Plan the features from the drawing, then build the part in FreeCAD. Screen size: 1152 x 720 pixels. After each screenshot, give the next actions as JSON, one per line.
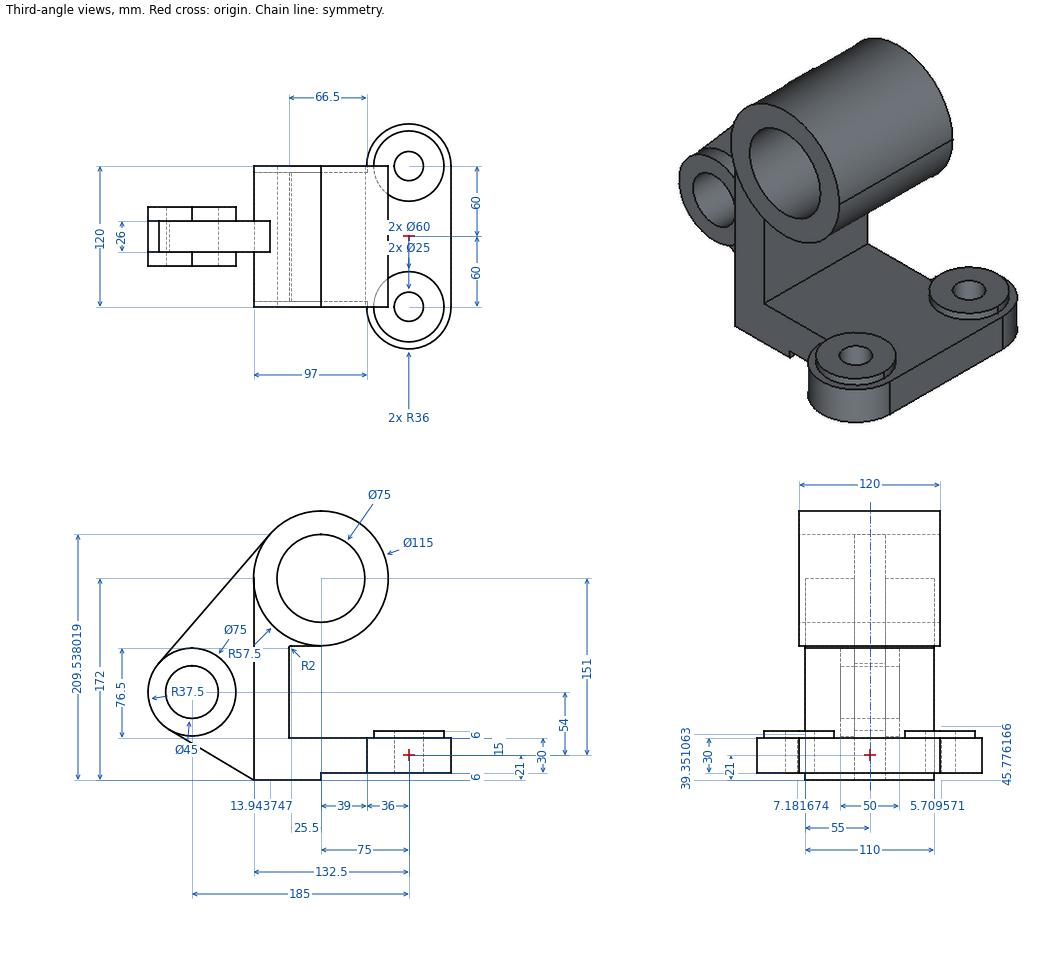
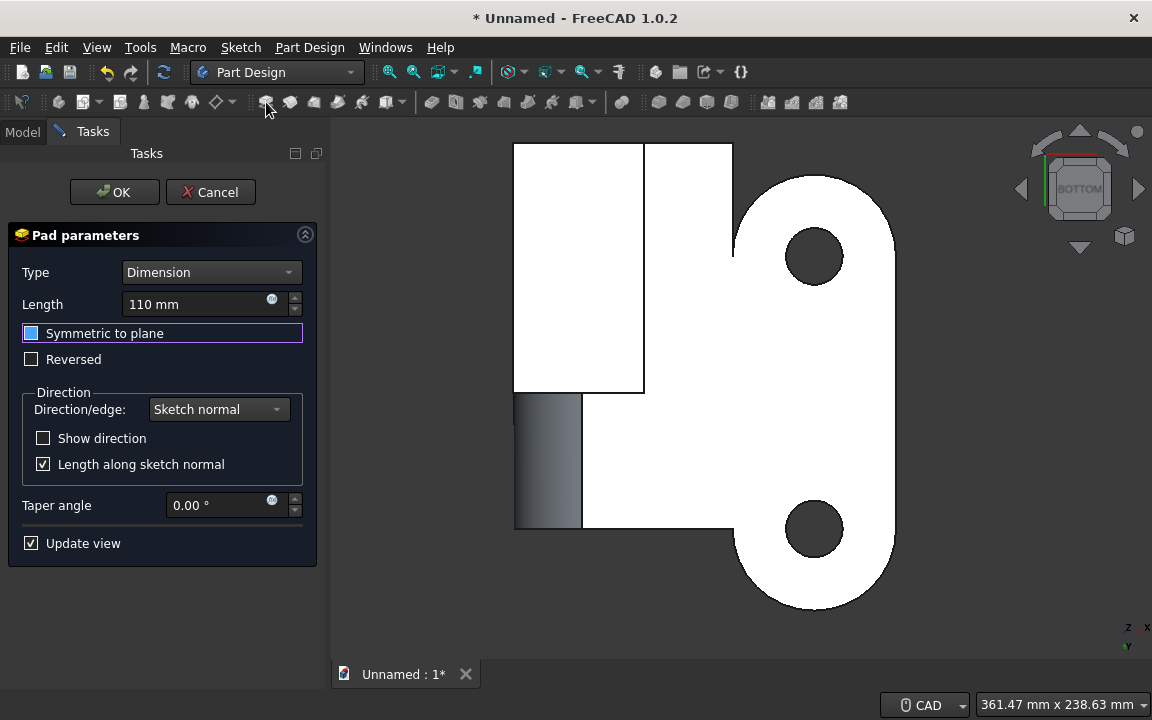
{"action": "left_click", "coordinate": [30, 333]}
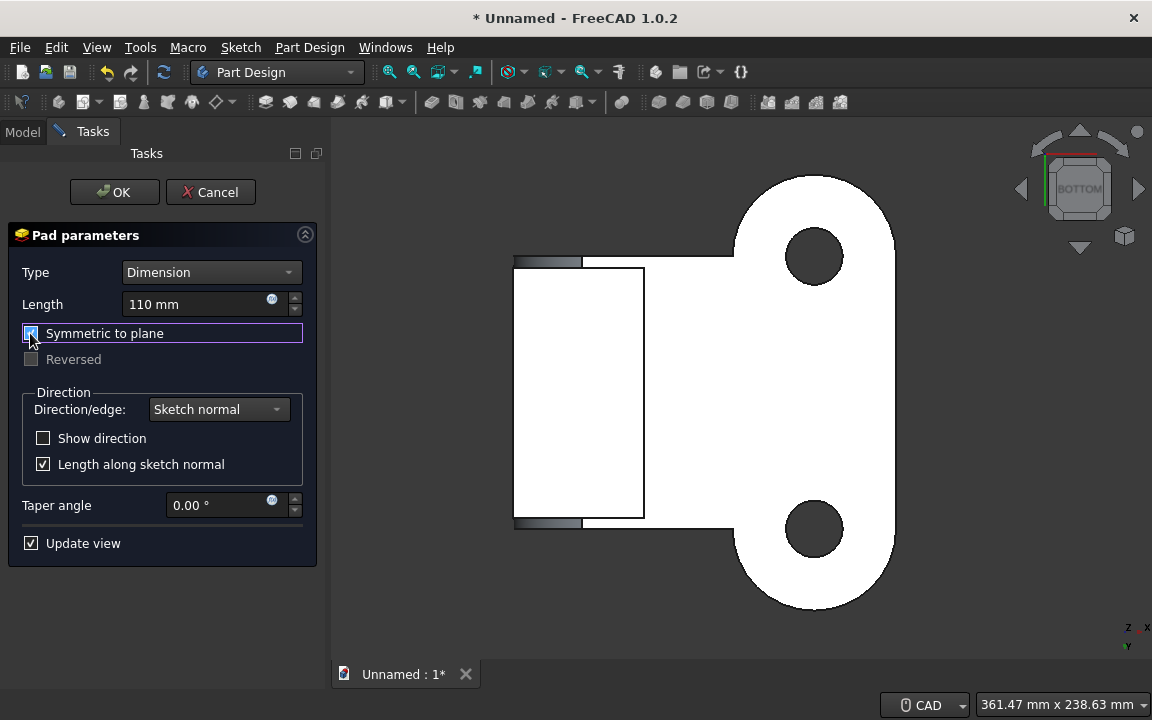
{"action": "left_click", "coordinate": [115, 192]}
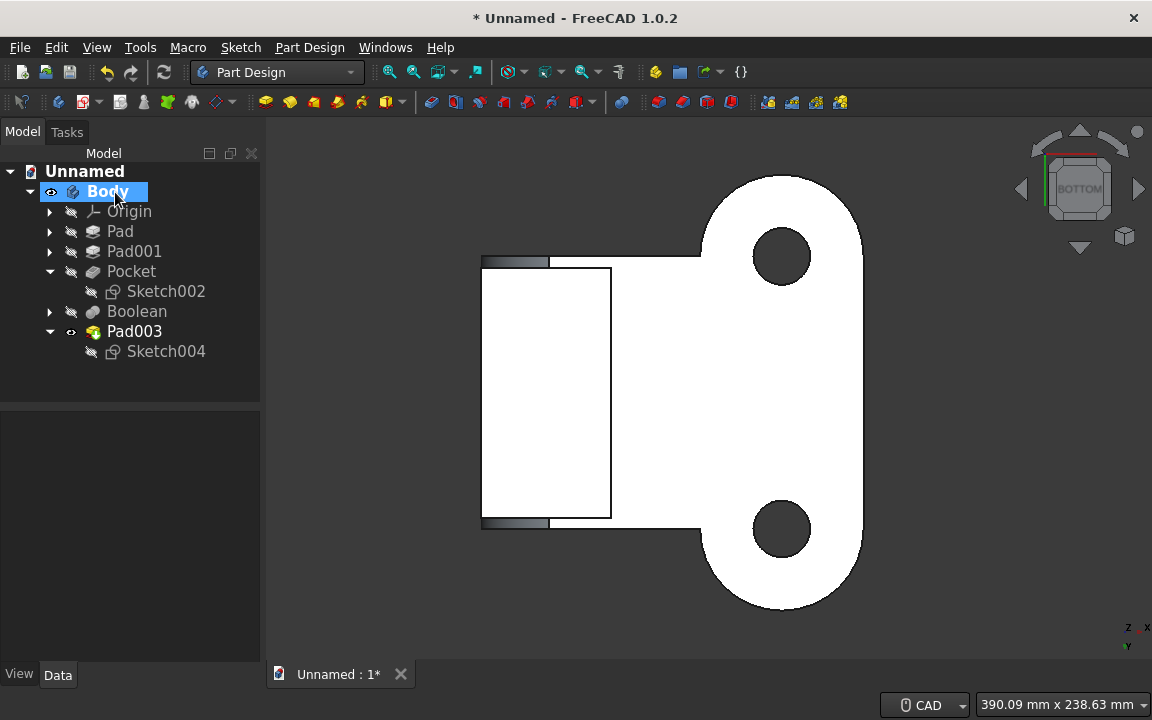
{"action": "key", "text": "6"}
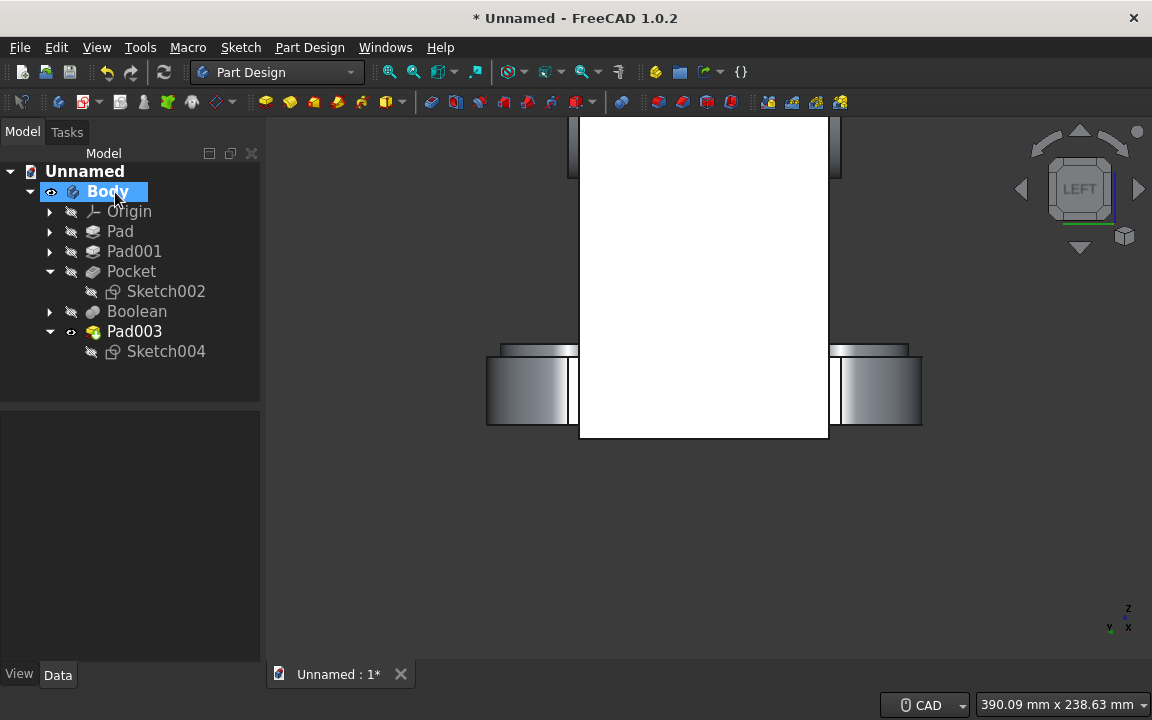
{"action": "key", "text": "v f"}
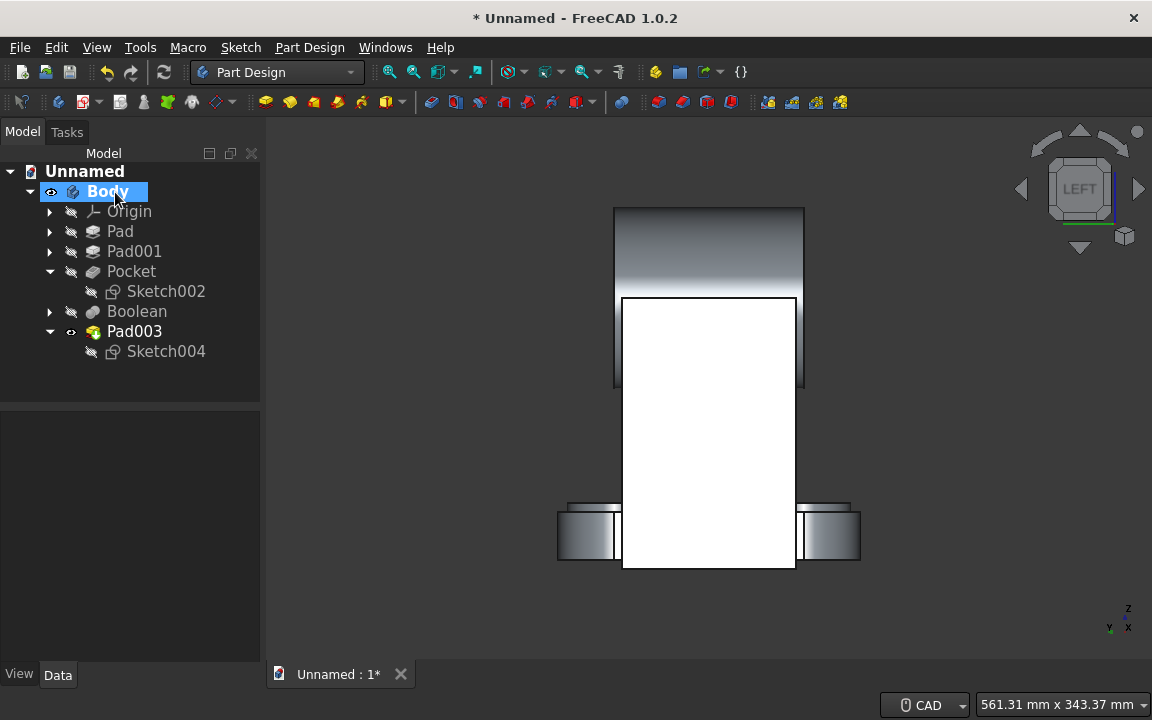
{"action": "left_click", "coordinate": [709, 394]}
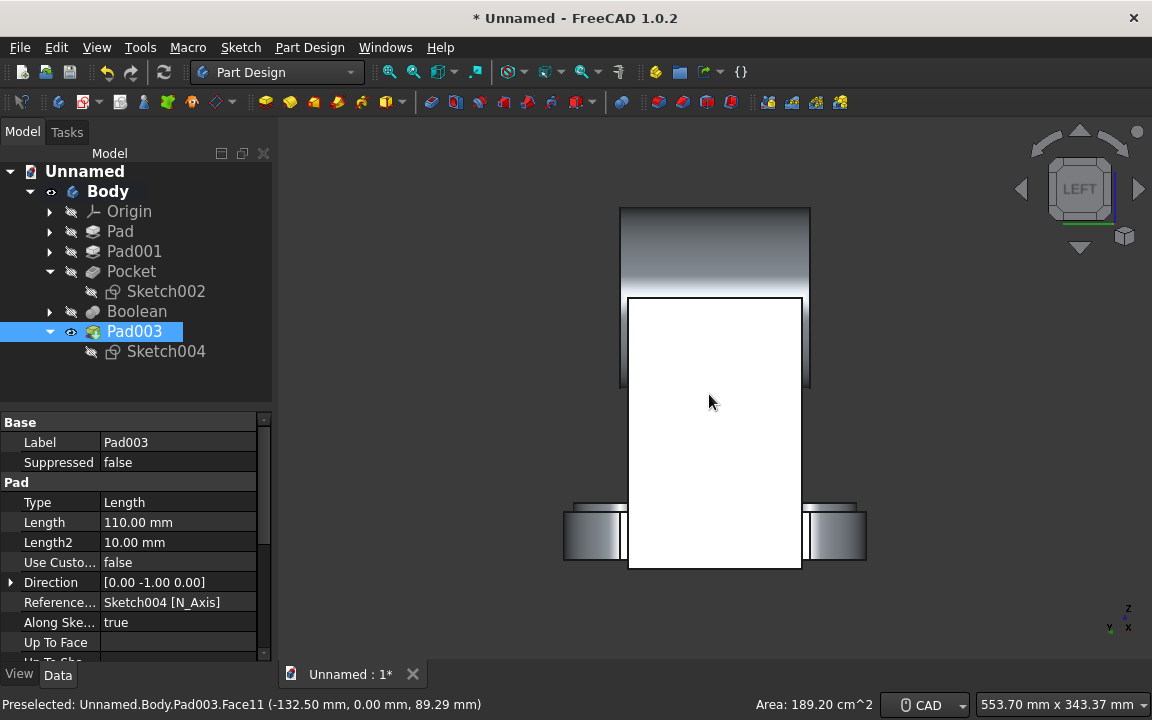
{"action": "left_click", "coordinate": [84, 102]}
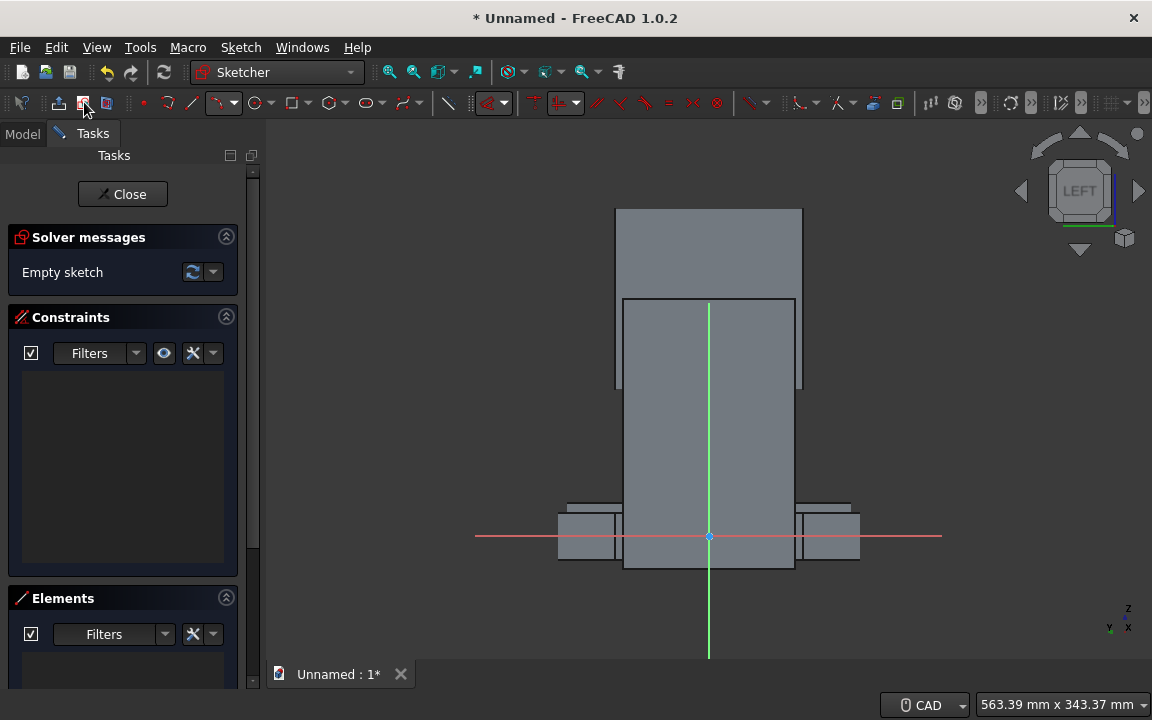
{"action": "scroll", "coordinate": [751, 617], "scroll_direction": "up", "scroll_amount": 5}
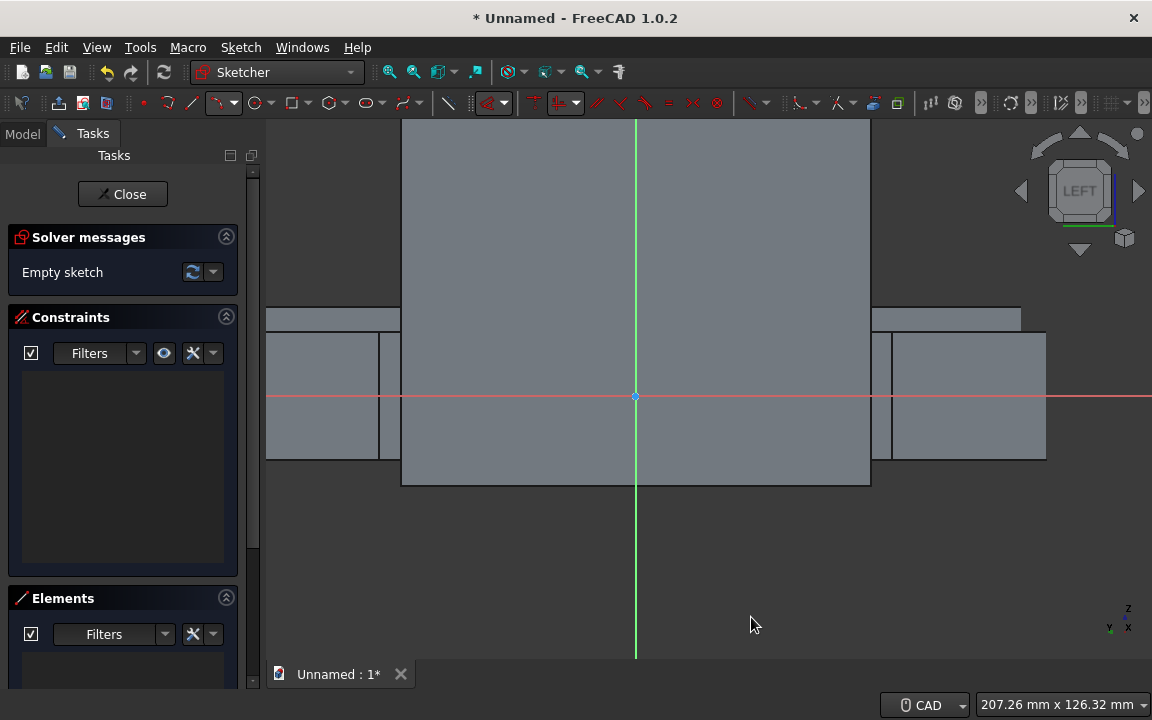
{"action": "key", "text": "g r"}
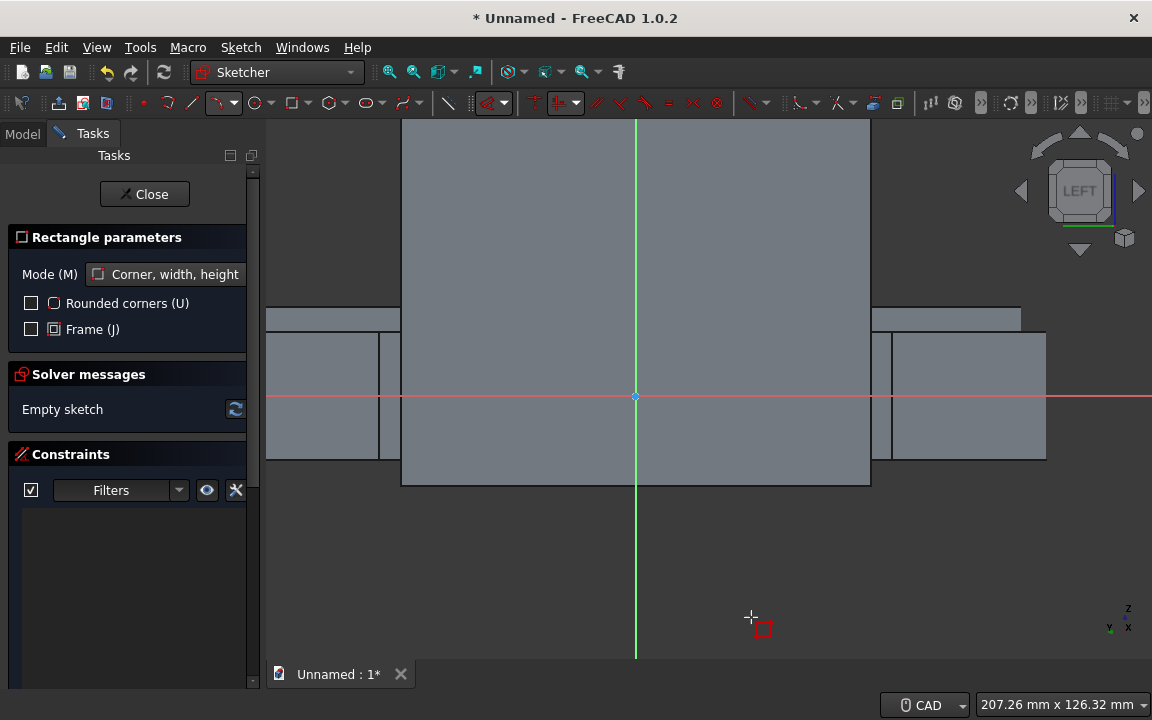
{"action": "left_click", "coordinate": [871, 318]}
{"action": "left_click", "coordinate": [902, 486]}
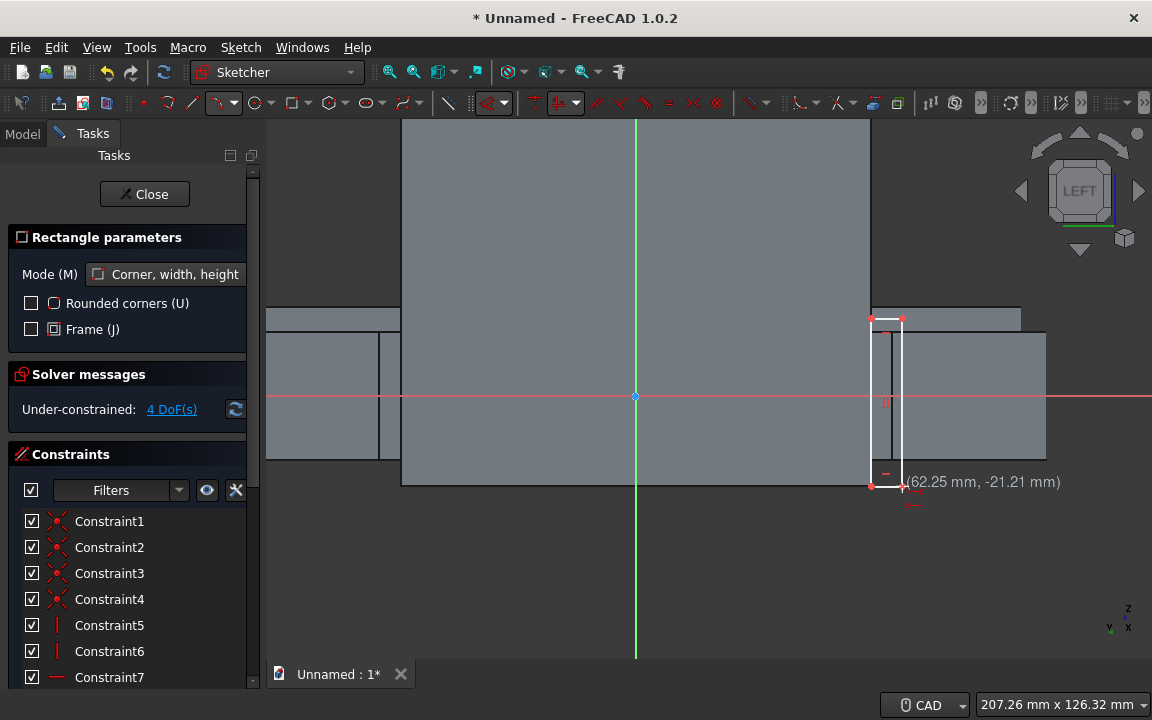
{"action": "left_click", "coordinate": [376, 290]}
{"action": "left_click", "coordinate": [401, 486]}
{"action": "key", "text": "Escape"}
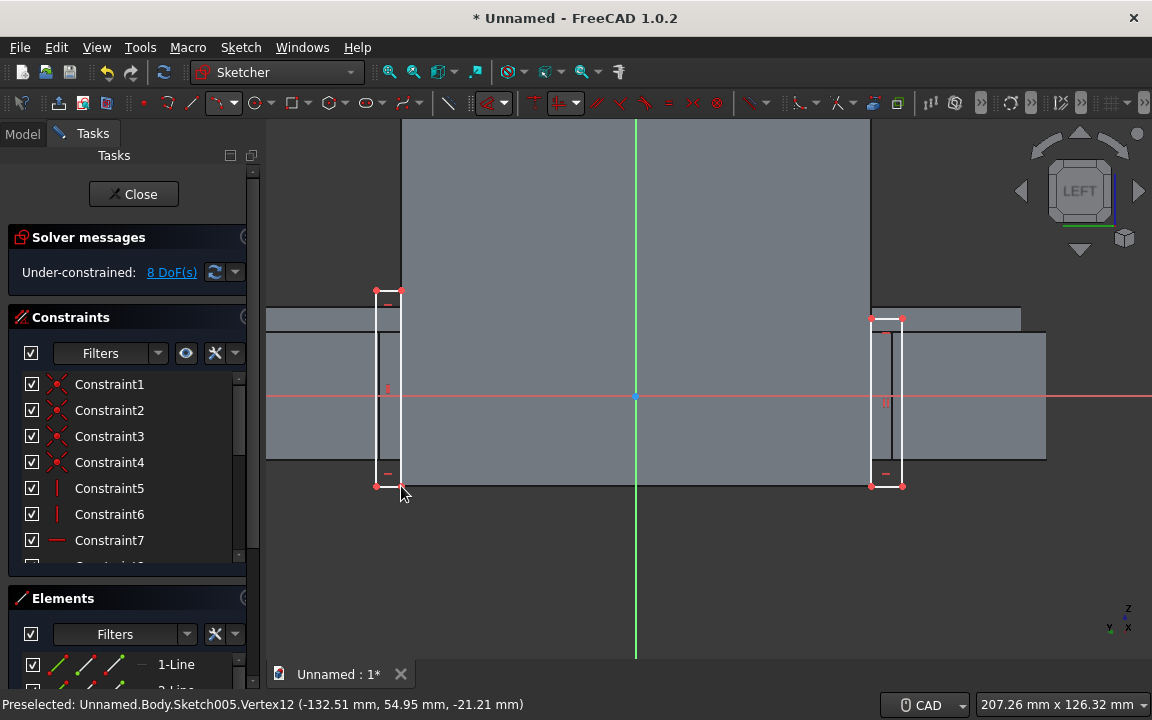
{"action": "left_click", "coordinate": [871, 487]}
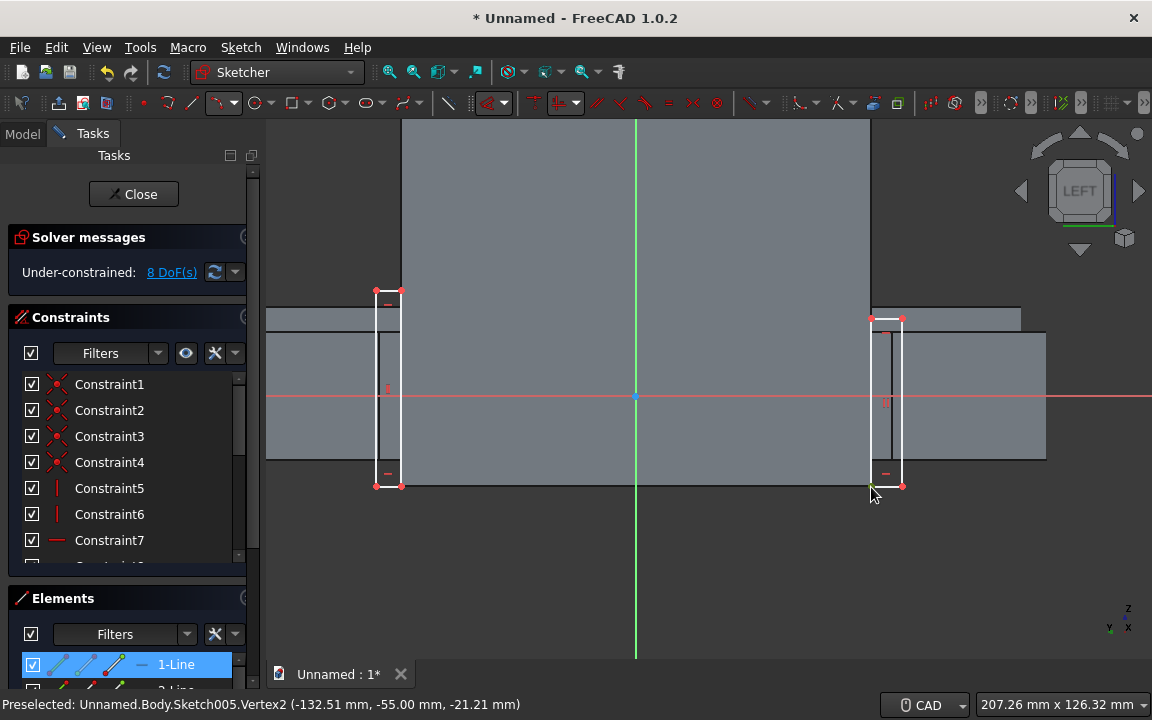
{"action": "left_click", "coordinate": [401, 487]}